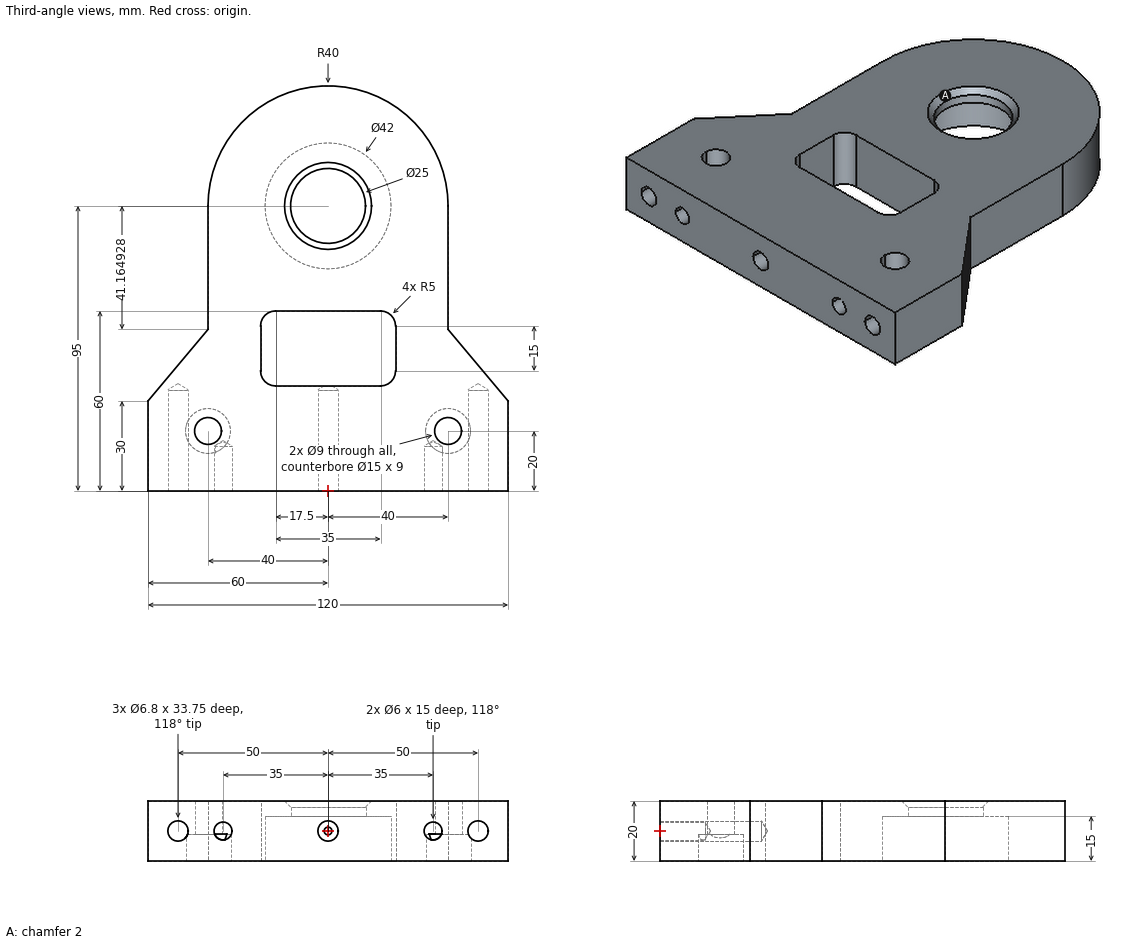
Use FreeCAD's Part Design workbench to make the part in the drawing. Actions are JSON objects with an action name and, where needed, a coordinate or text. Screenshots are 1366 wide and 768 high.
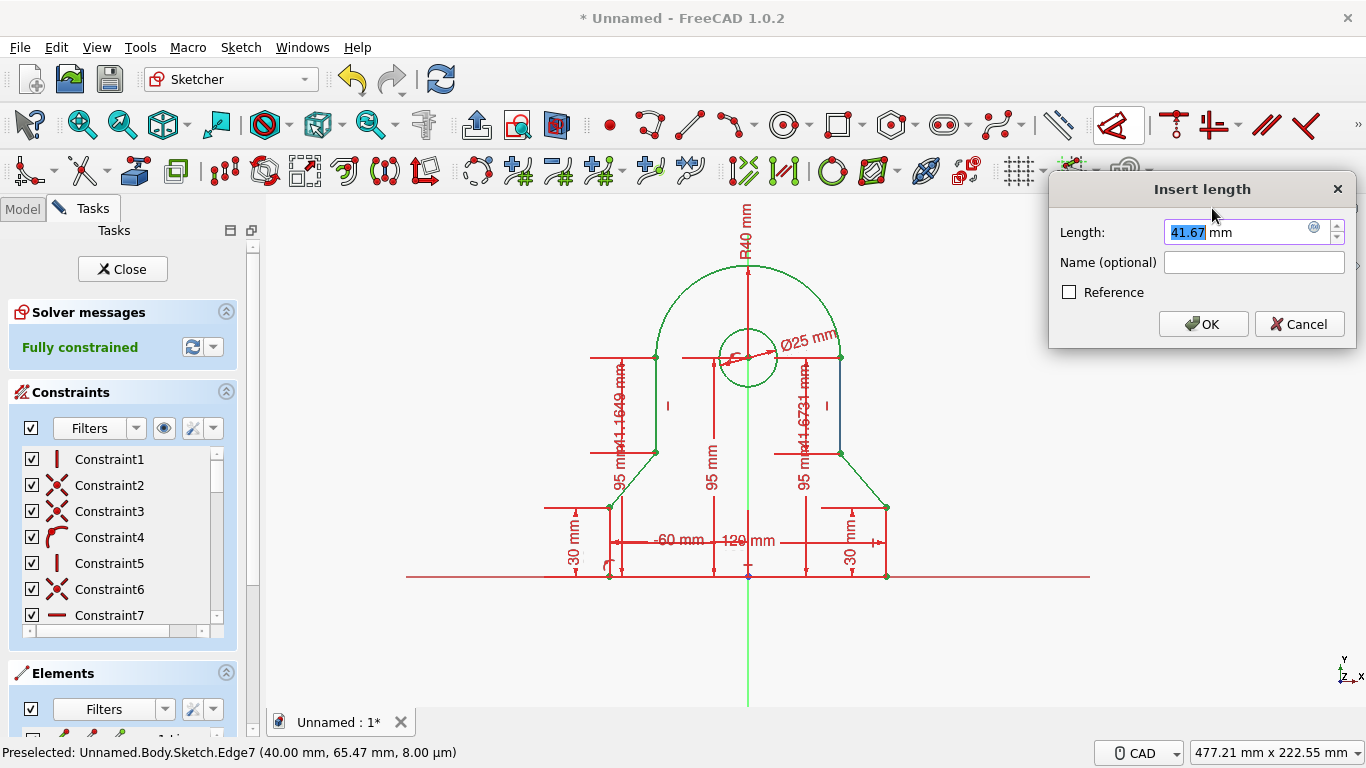
{"action": "type", "text": "41.164928"}
{"action": "key", "text": "Return"}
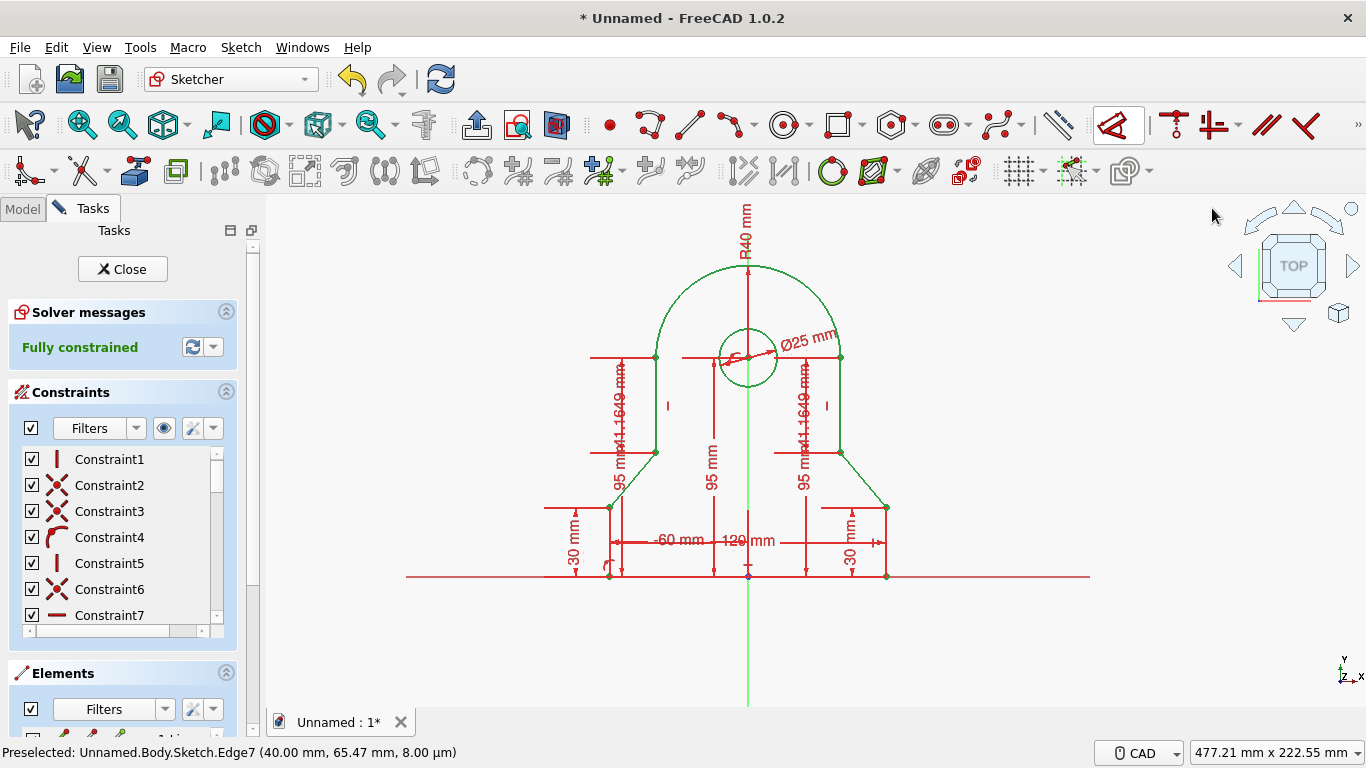
{"action": "left_click", "coordinate": [123, 269]}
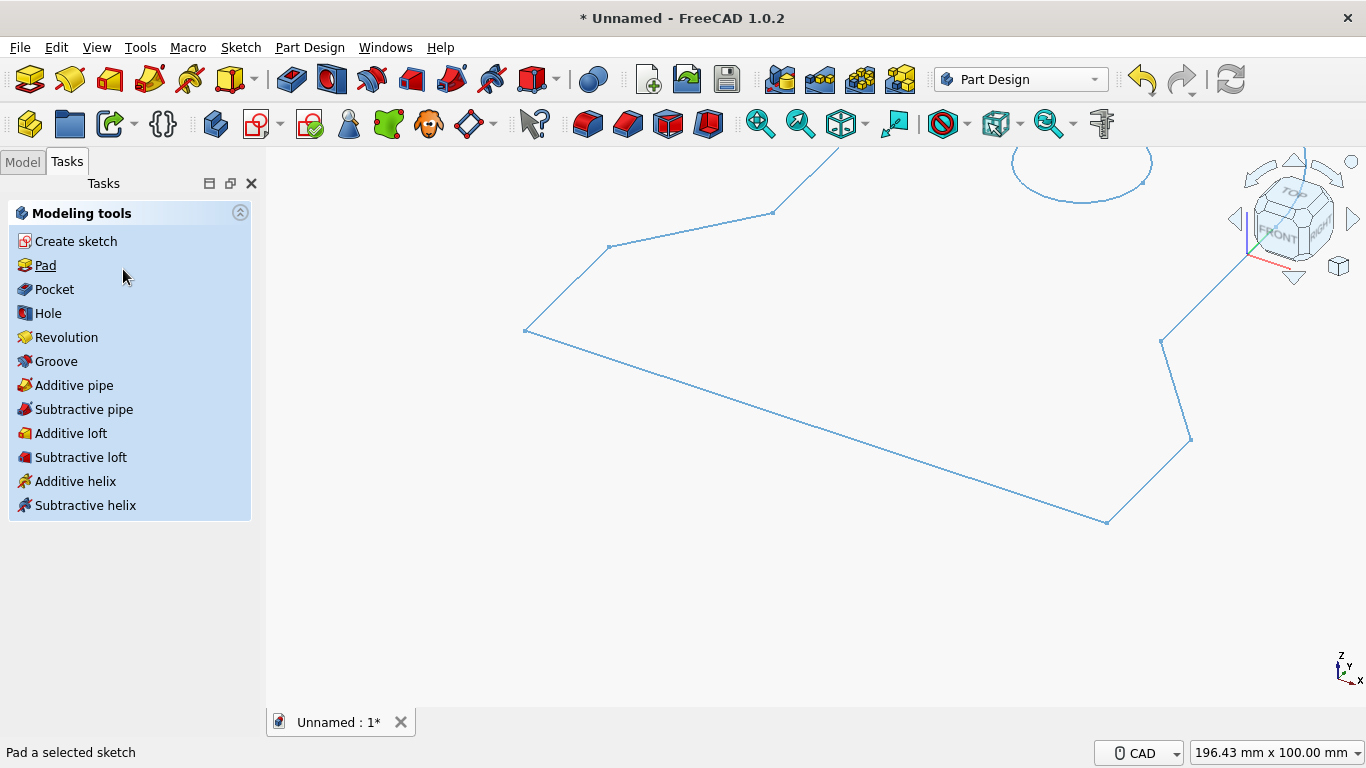
{"action": "left_click", "coordinate": [30, 80]}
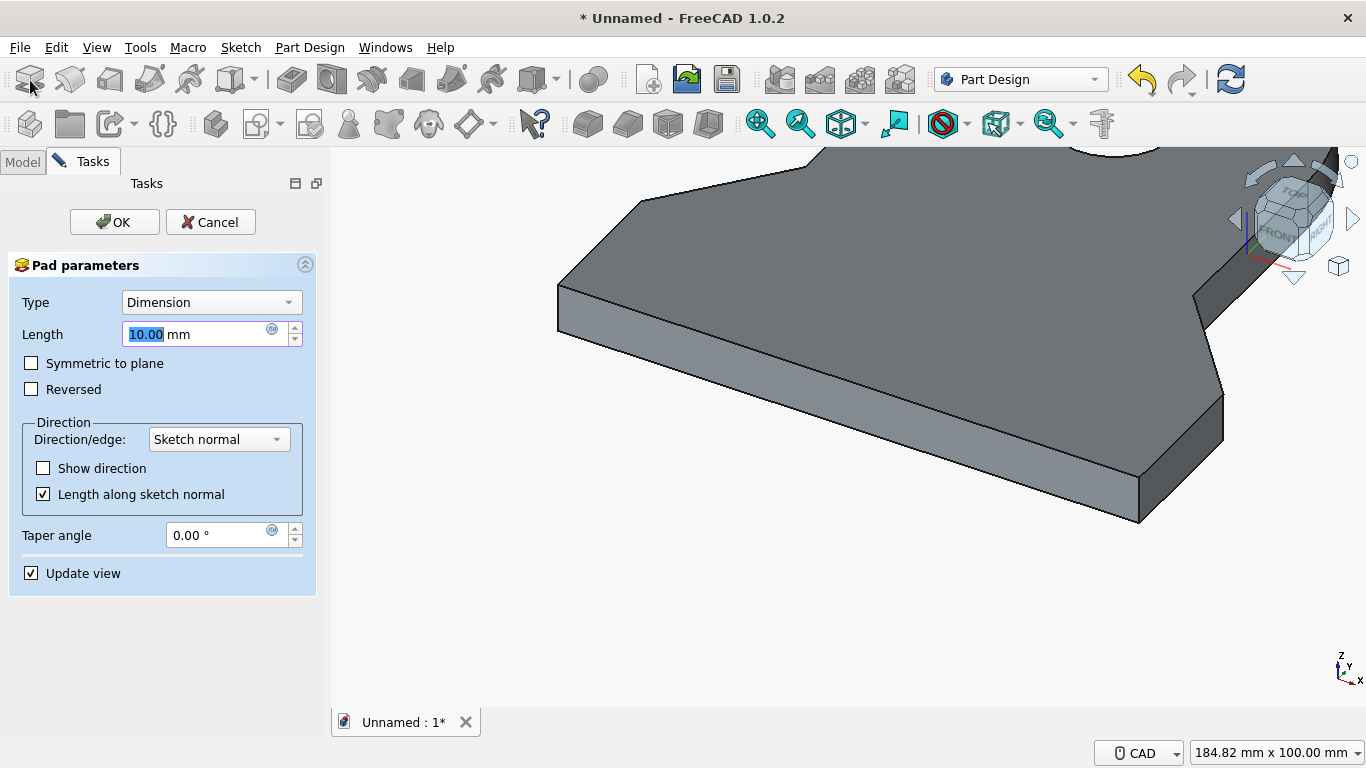
{"action": "type", "text": "20"}
{"action": "key", "text": "Tab"}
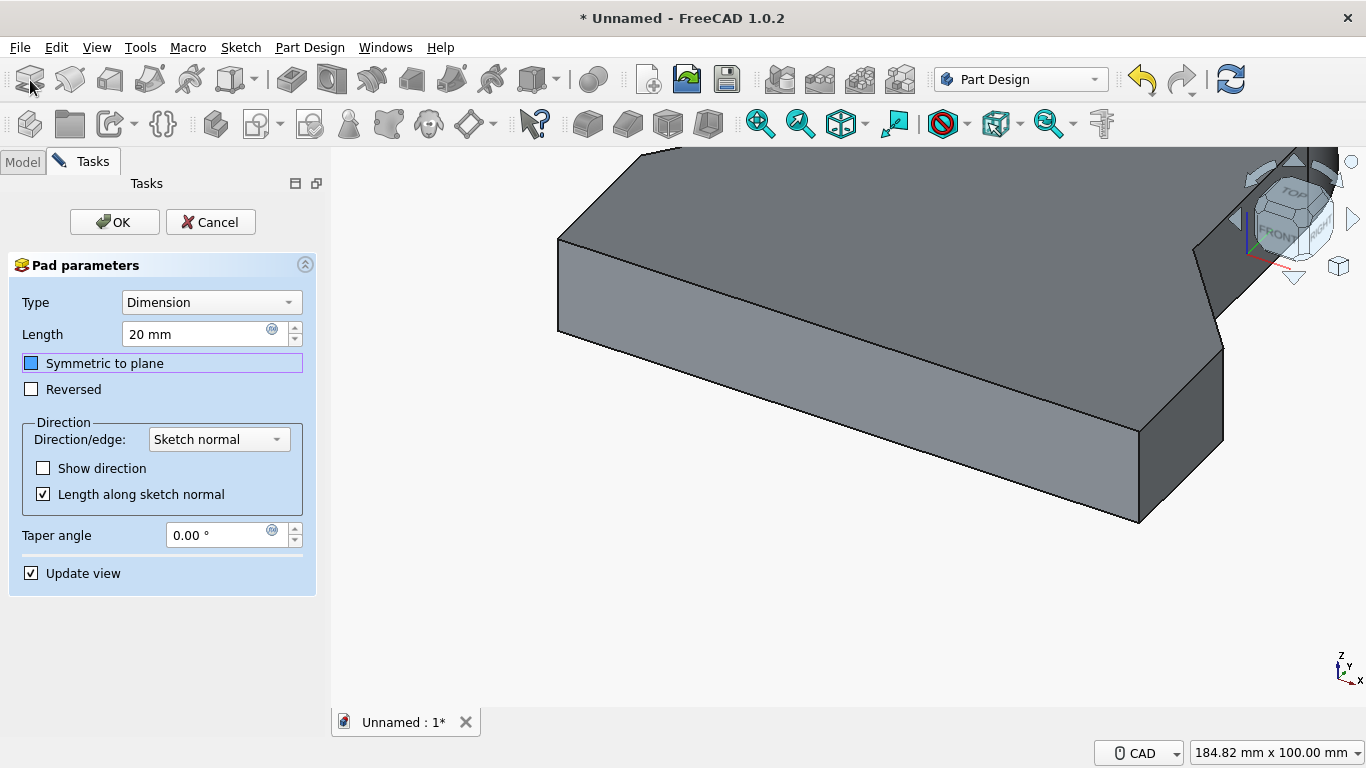
{"action": "left_click", "coordinate": [30, 363]}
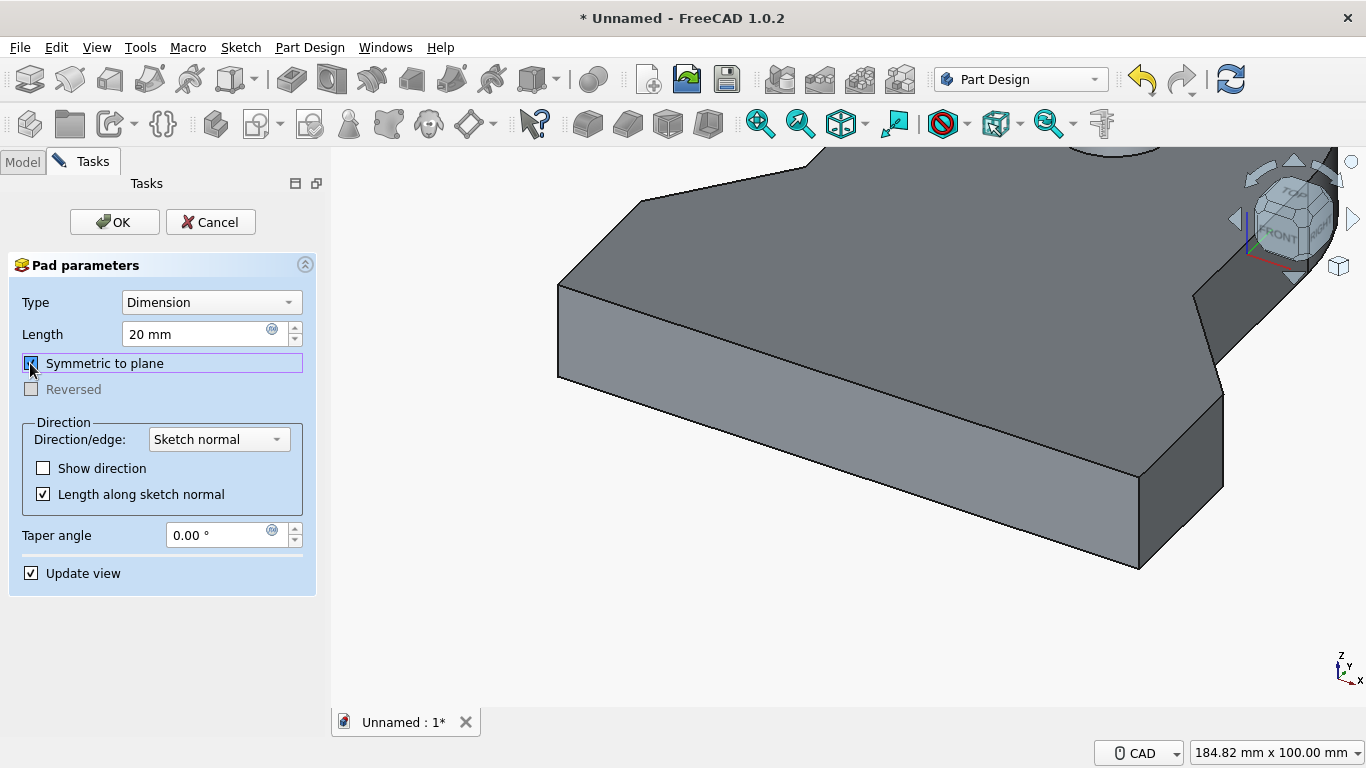
{"action": "left_click", "coordinate": [115, 222]}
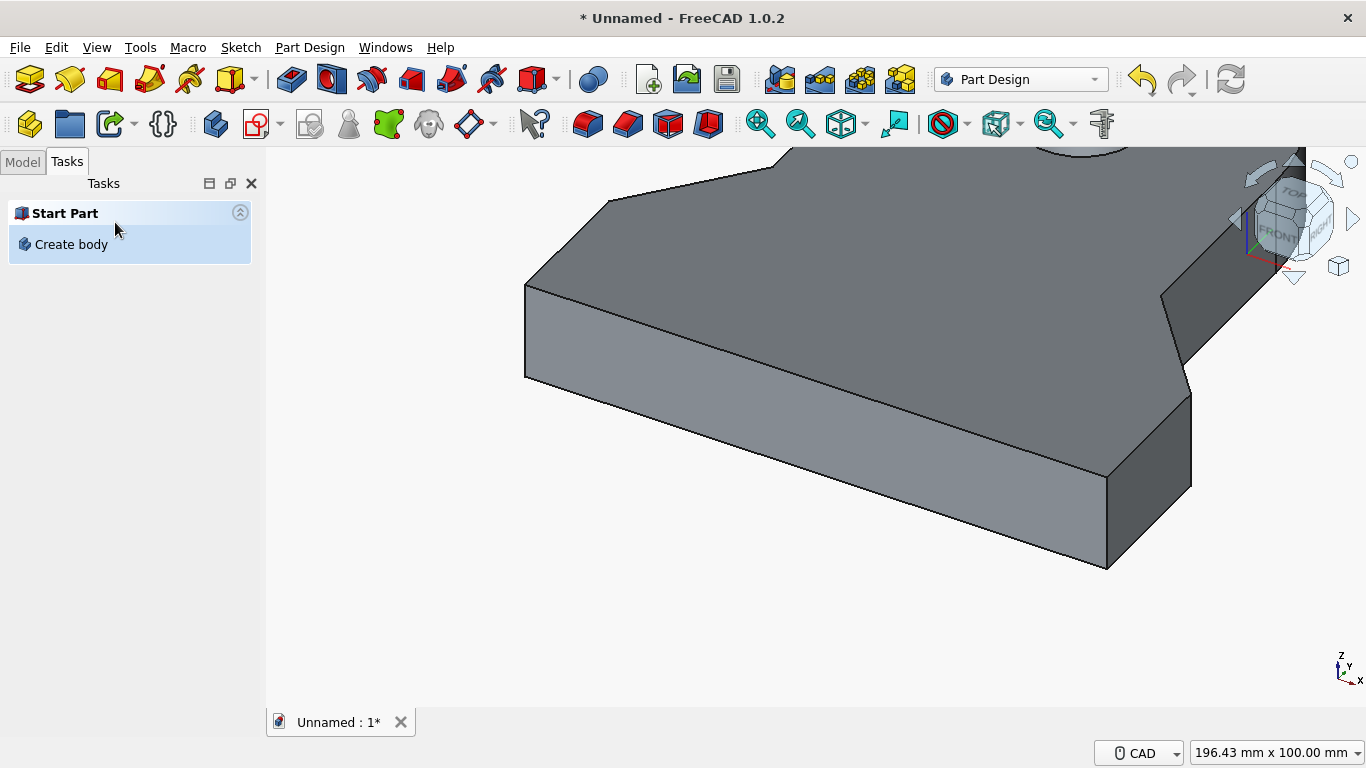
{"action": "left_click", "coordinate": [762, 124]}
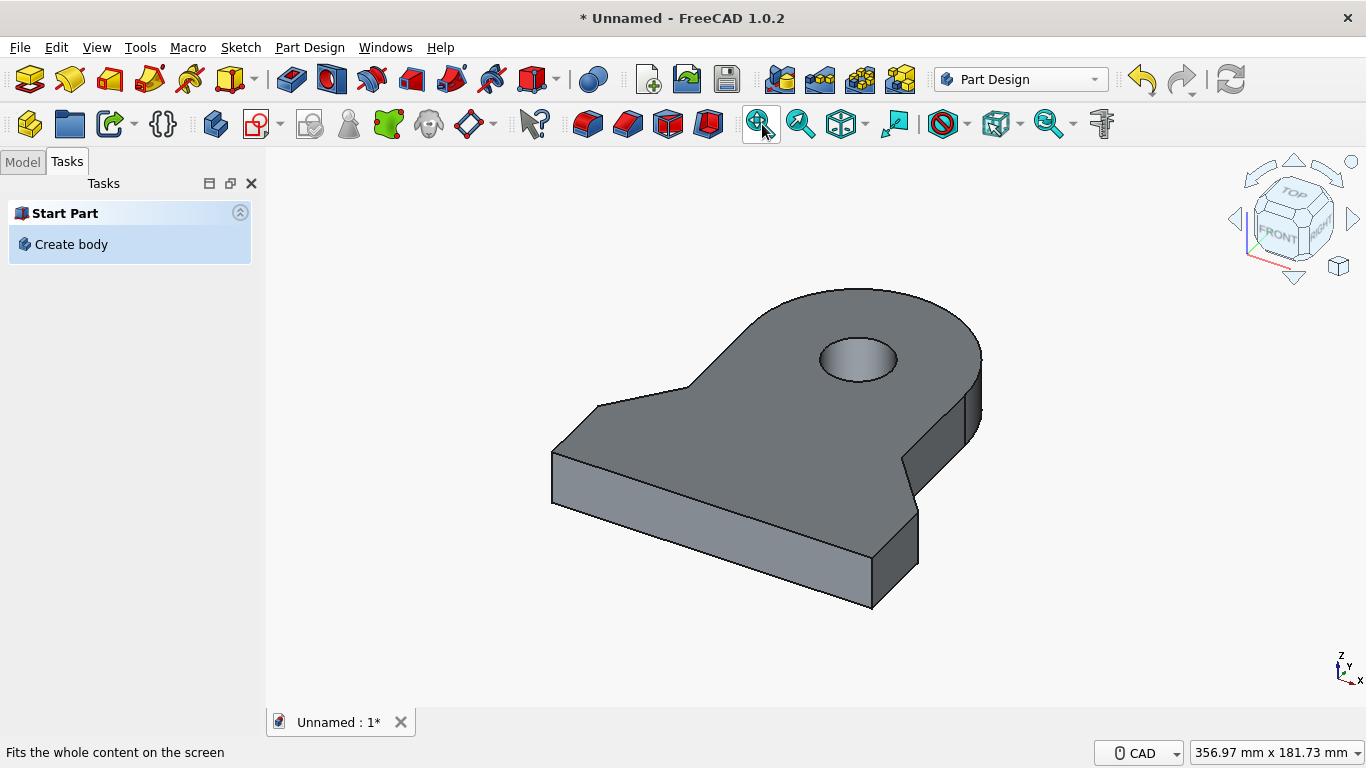
{"action": "left_click", "coordinate": [256, 124]}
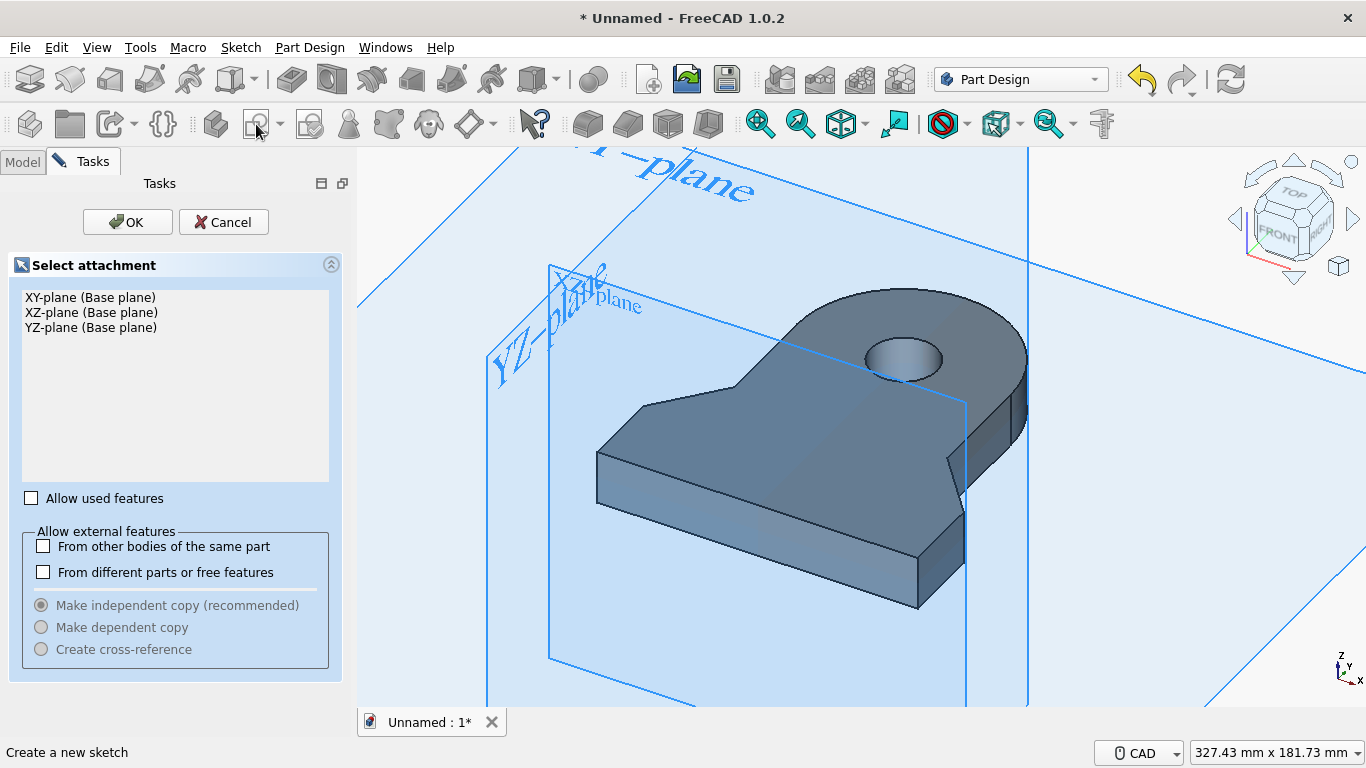
{"action": "left_click", "coordinate": [82, 312]}